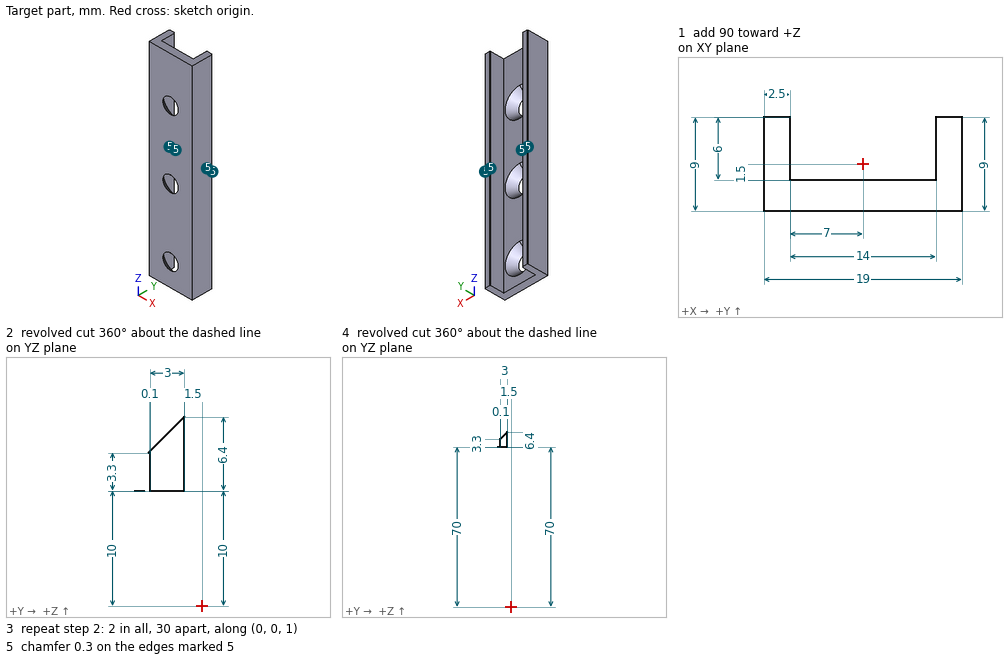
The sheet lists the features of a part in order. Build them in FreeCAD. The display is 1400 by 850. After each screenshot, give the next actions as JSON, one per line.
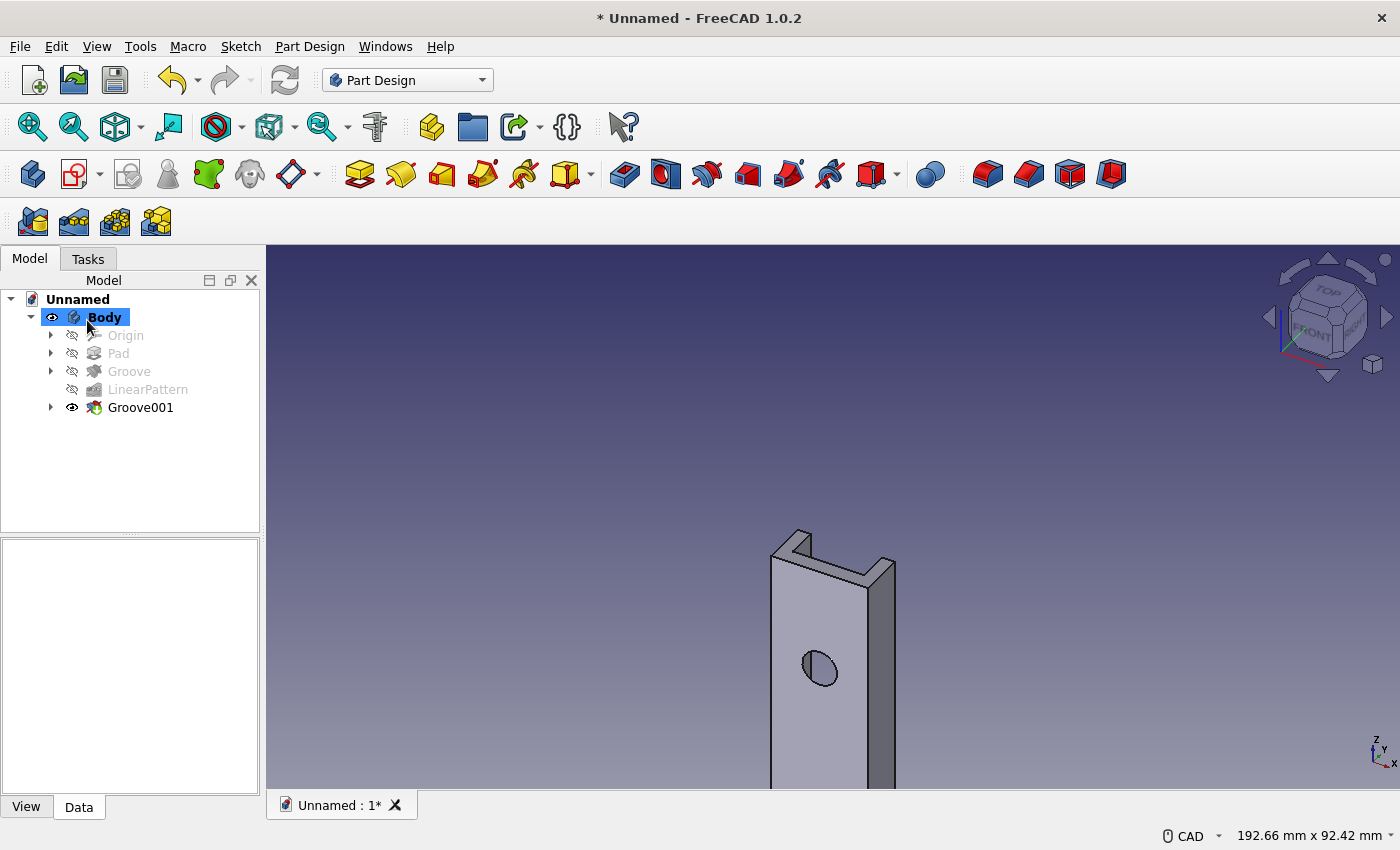
{"action": "left_click", "coordinate": [33, 128]}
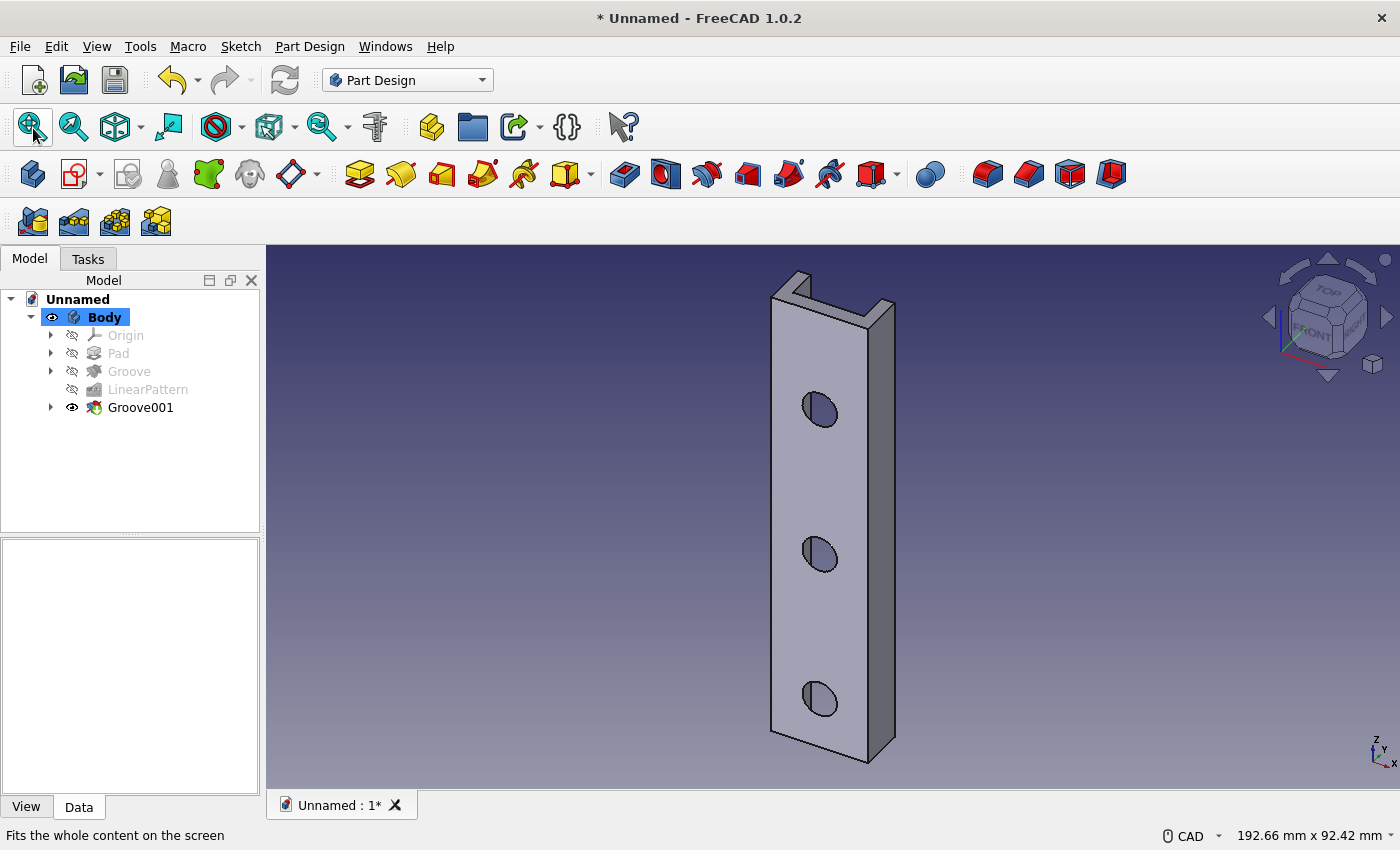
{"action": "key", "text": "0"}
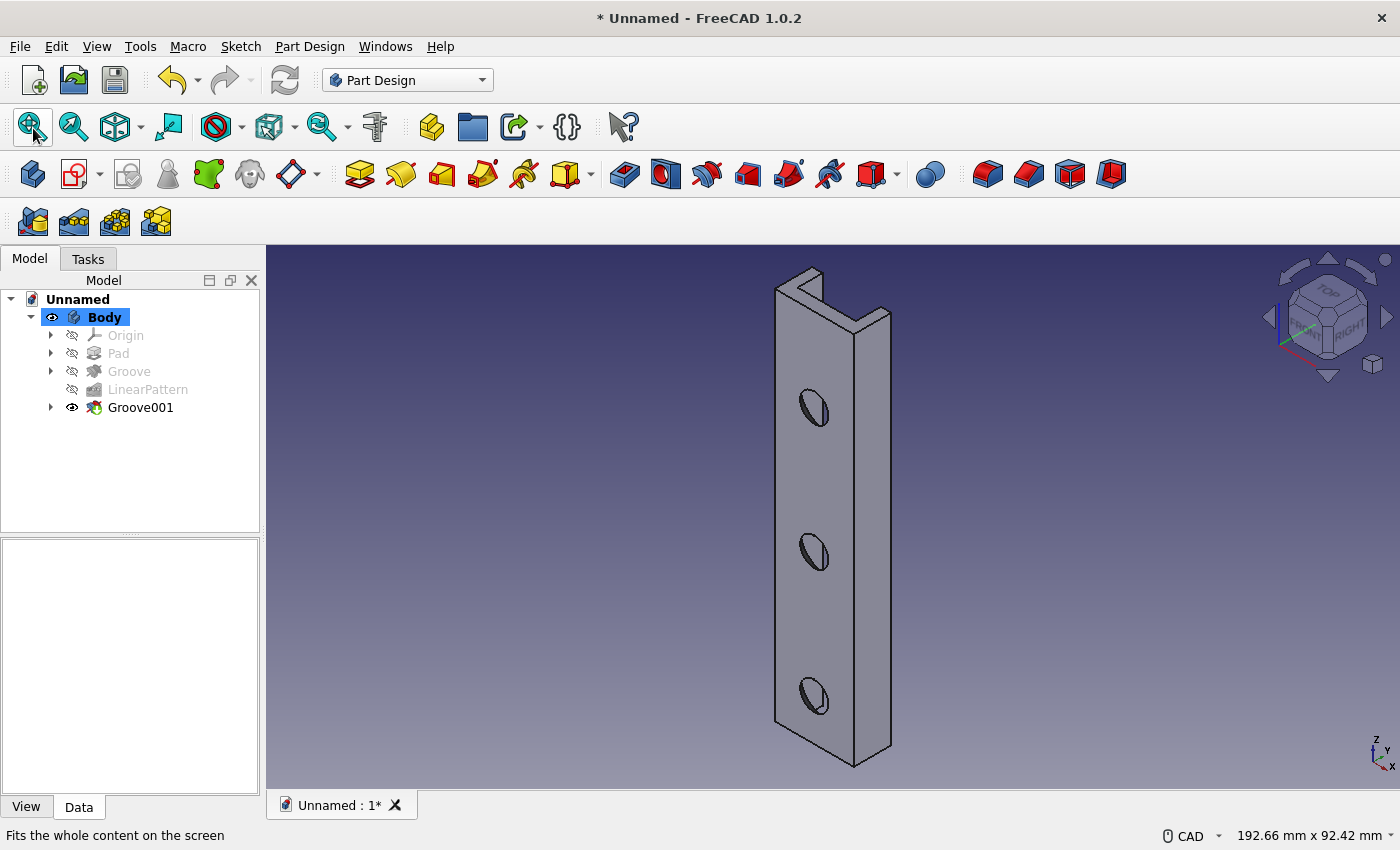
{"action": "key", "text": "2"}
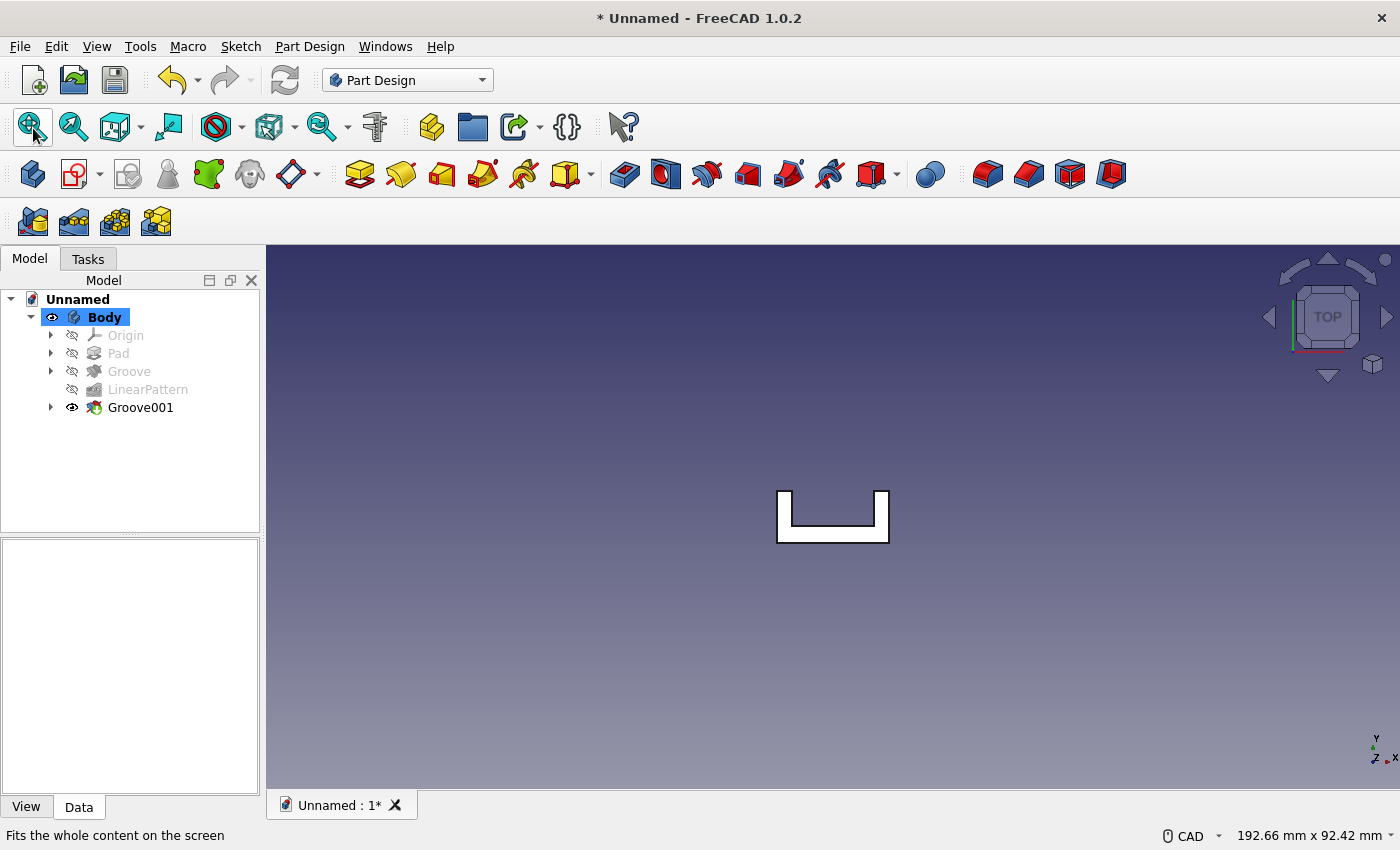
{"action": "left_click", "coordinate": [33, 128]}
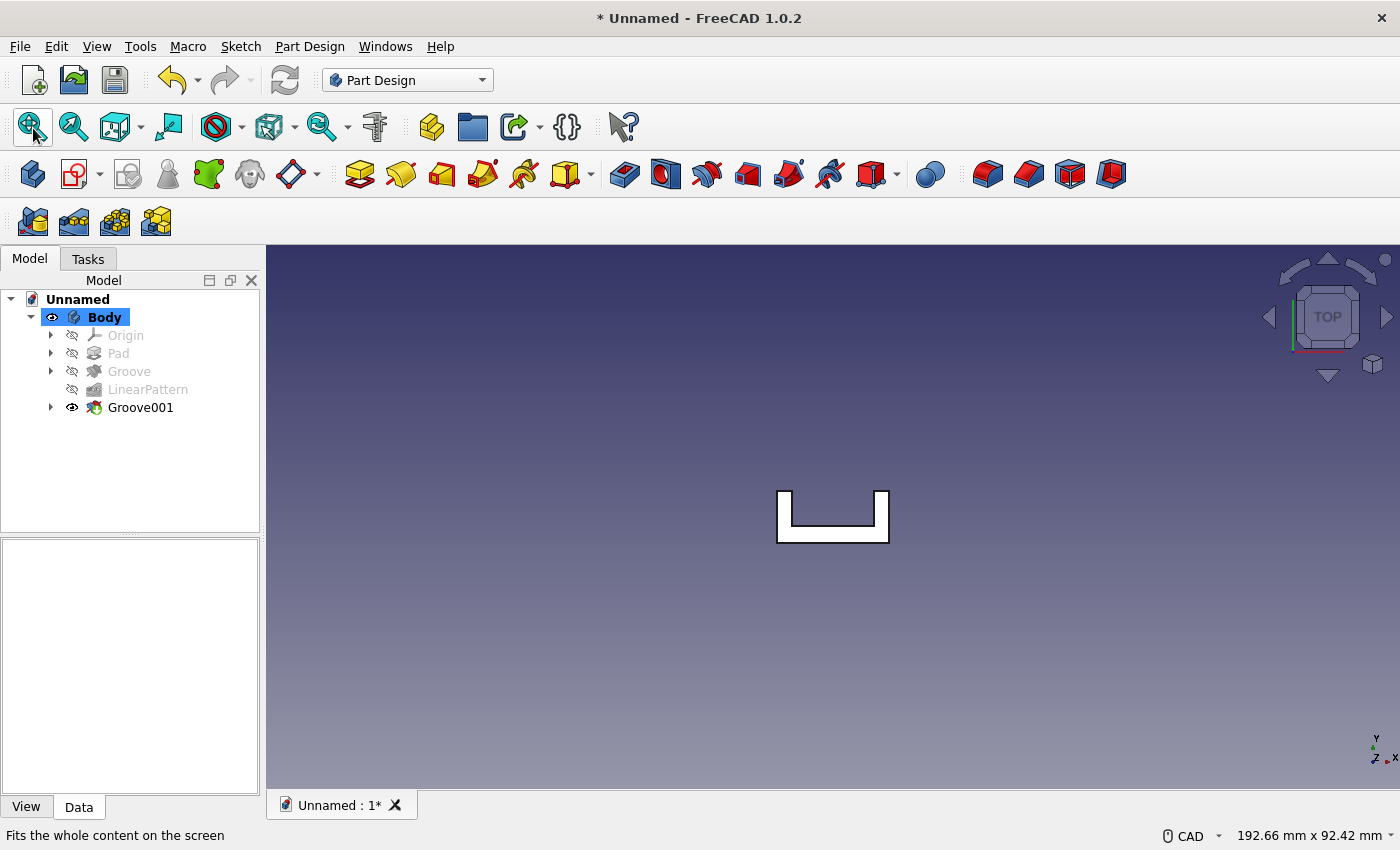
{"action": "key", "text": "1"}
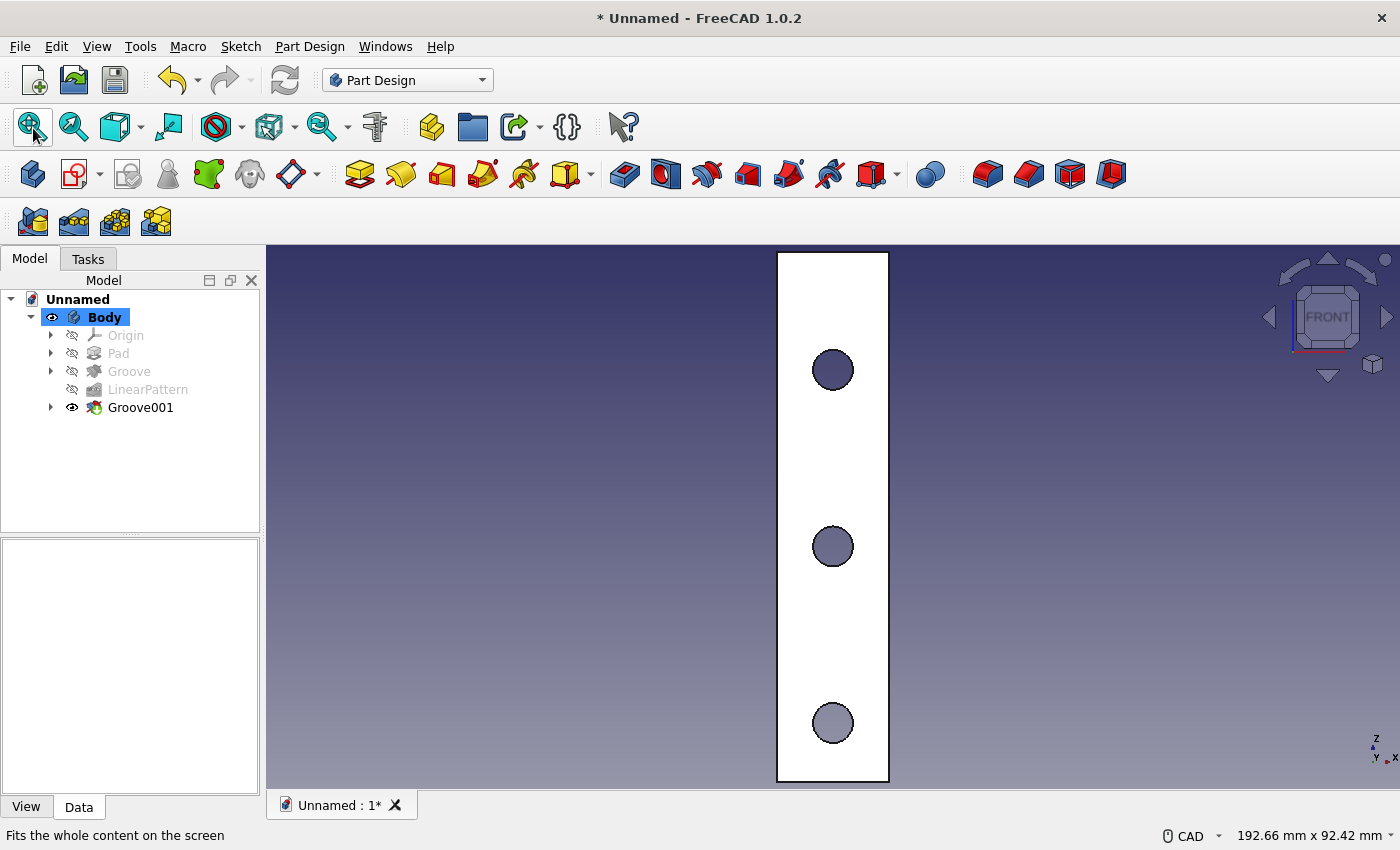
{"action": "key", "text": "3"}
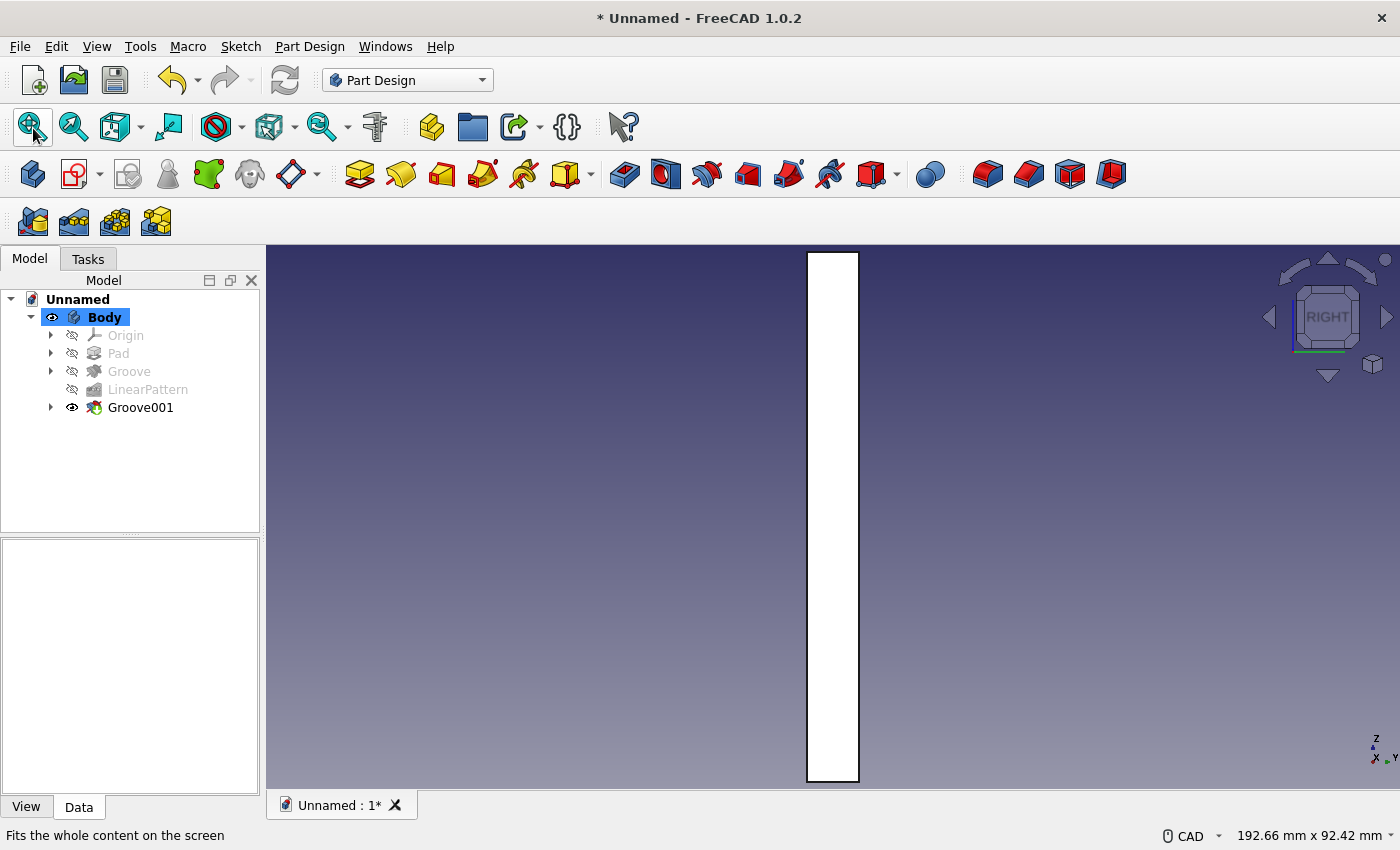
{"action": "left_click", "coordinate": [859, 516]}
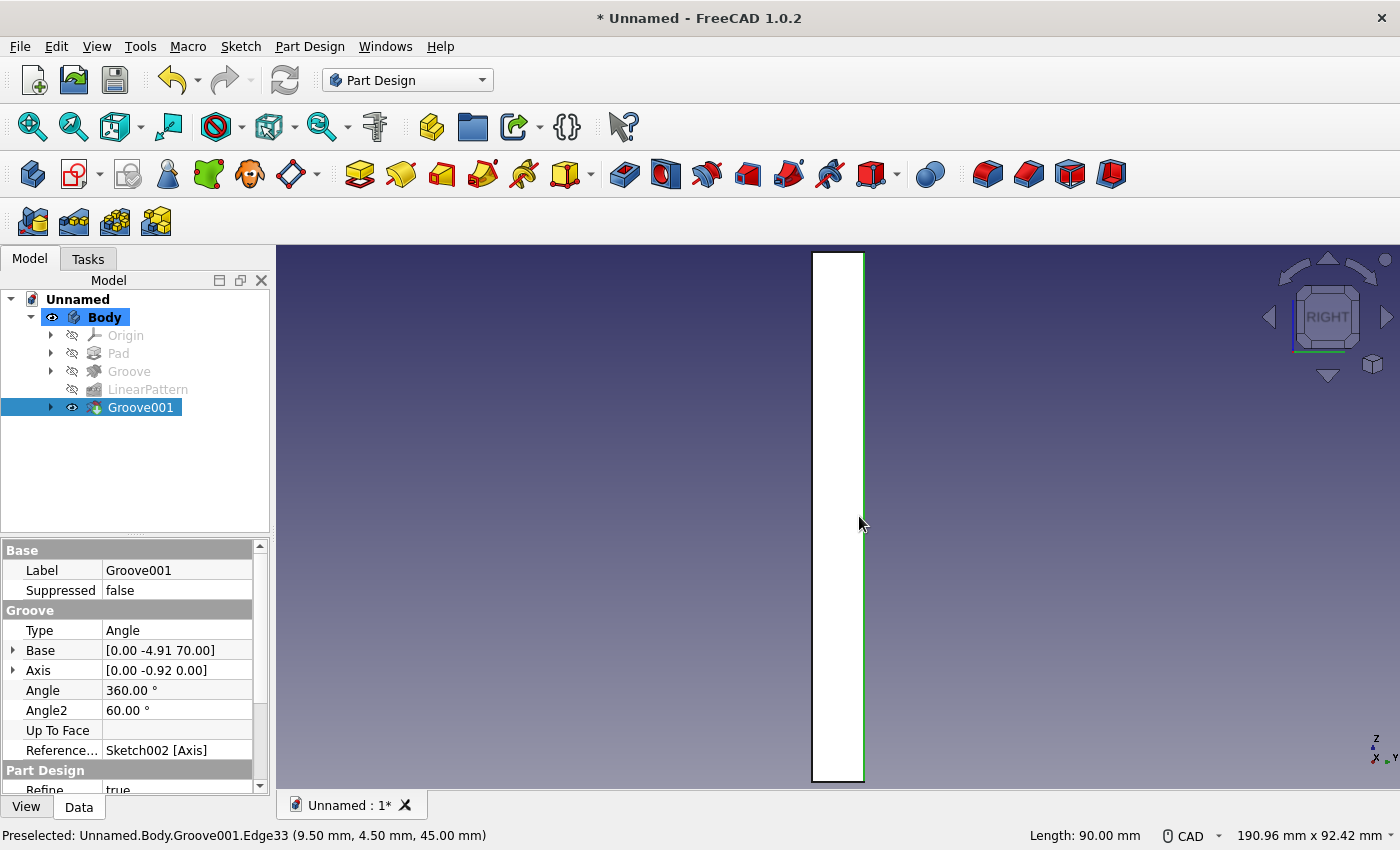
{"action": "key", "text": "5"}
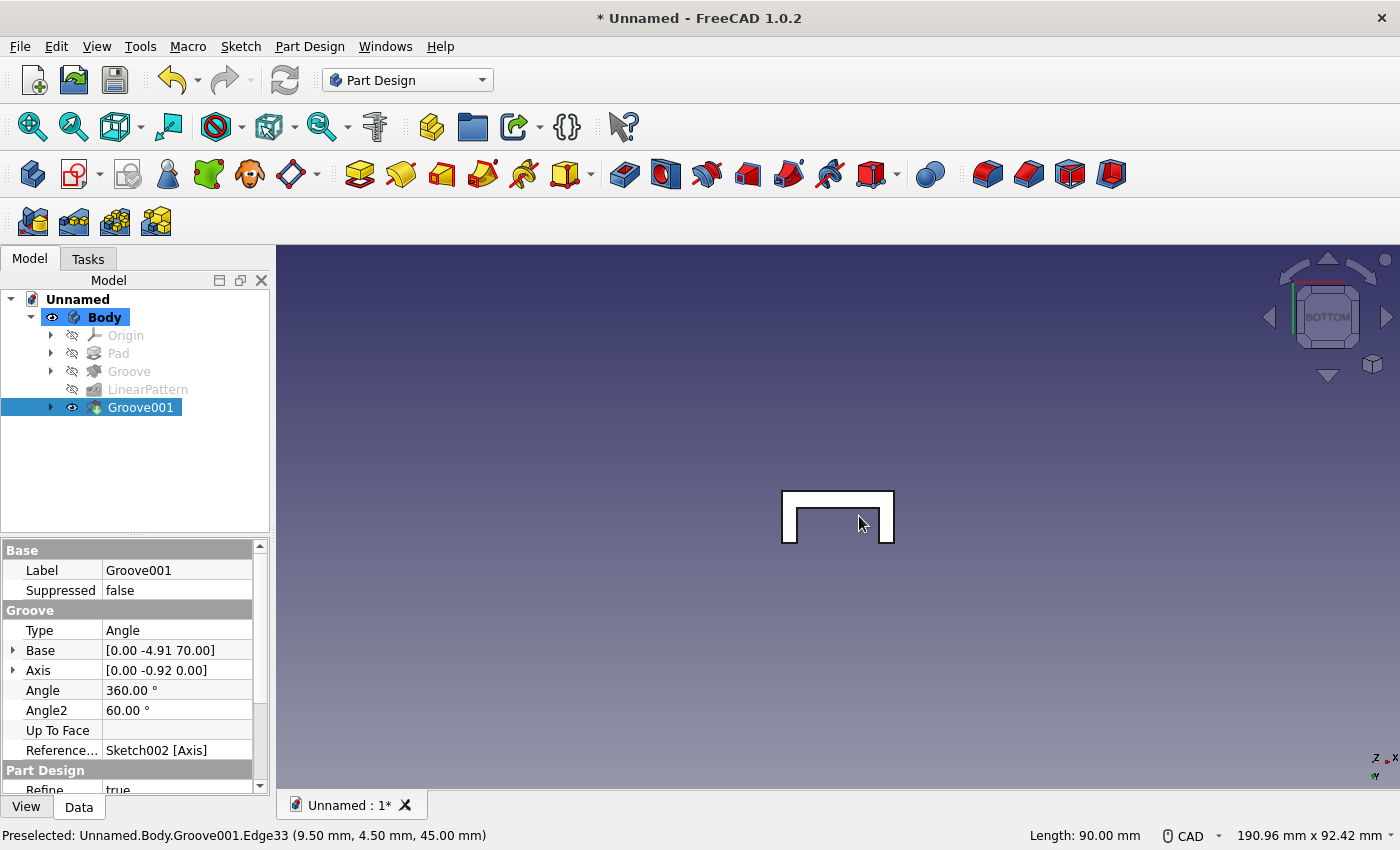
{"action": "left_click", "coordinate": [33, 128]}